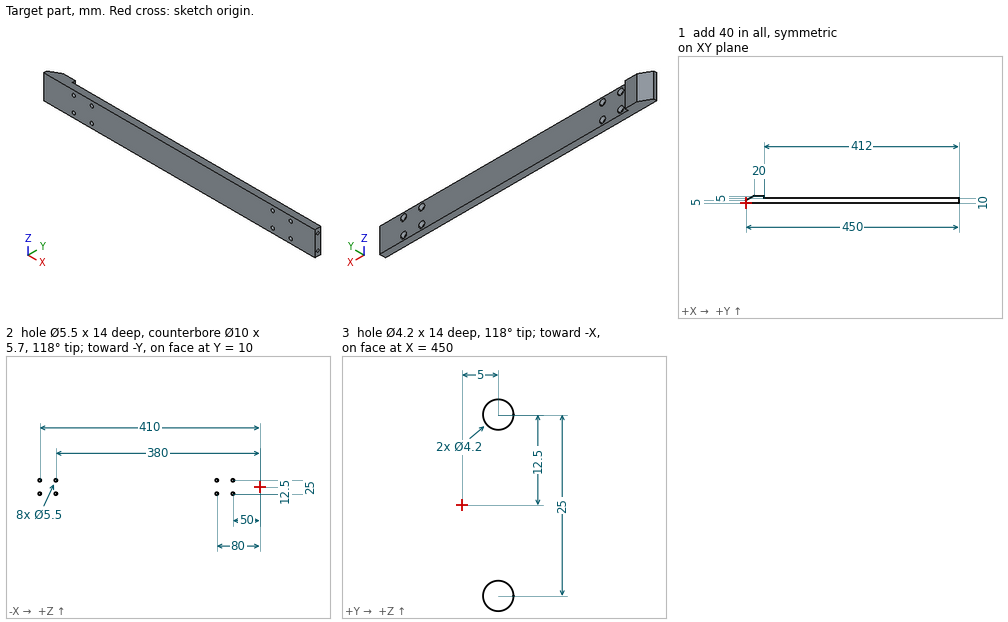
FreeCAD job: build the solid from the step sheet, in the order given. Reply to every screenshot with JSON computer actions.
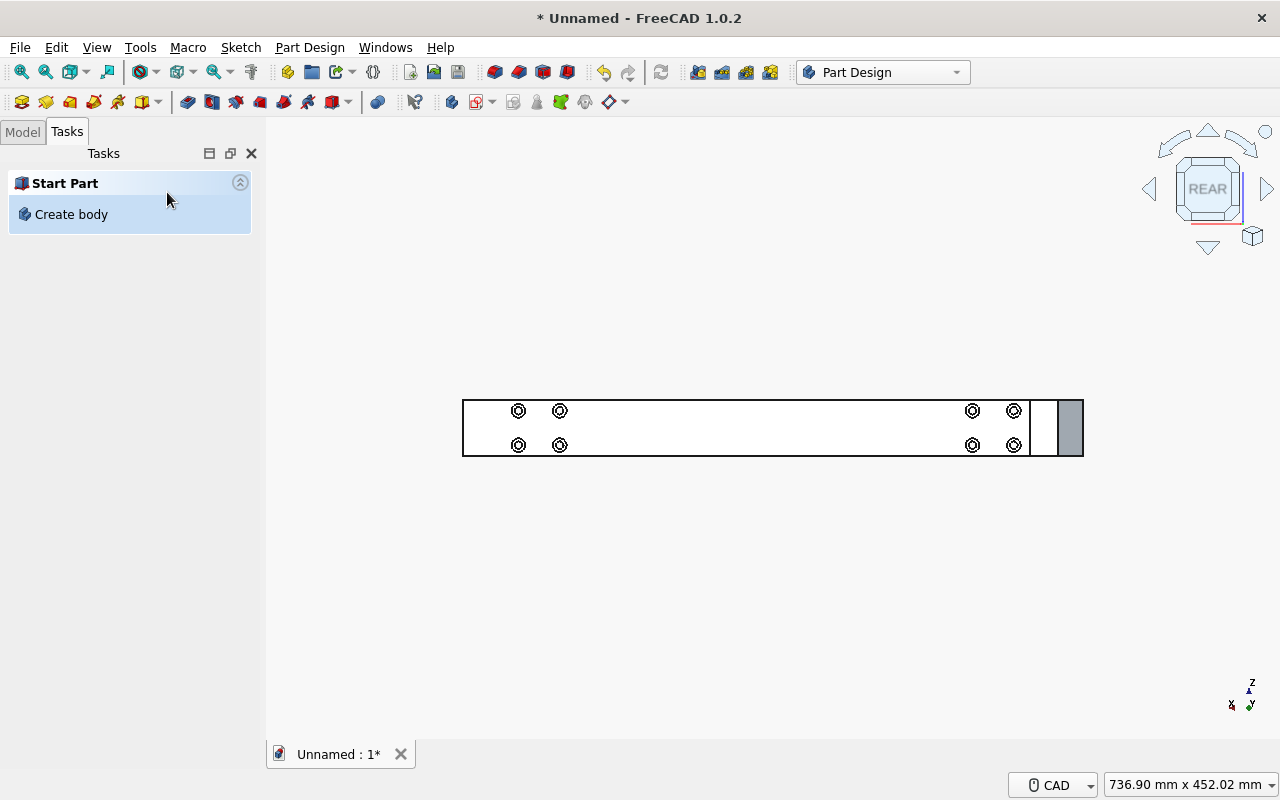
{"action": "key", "text": "0"}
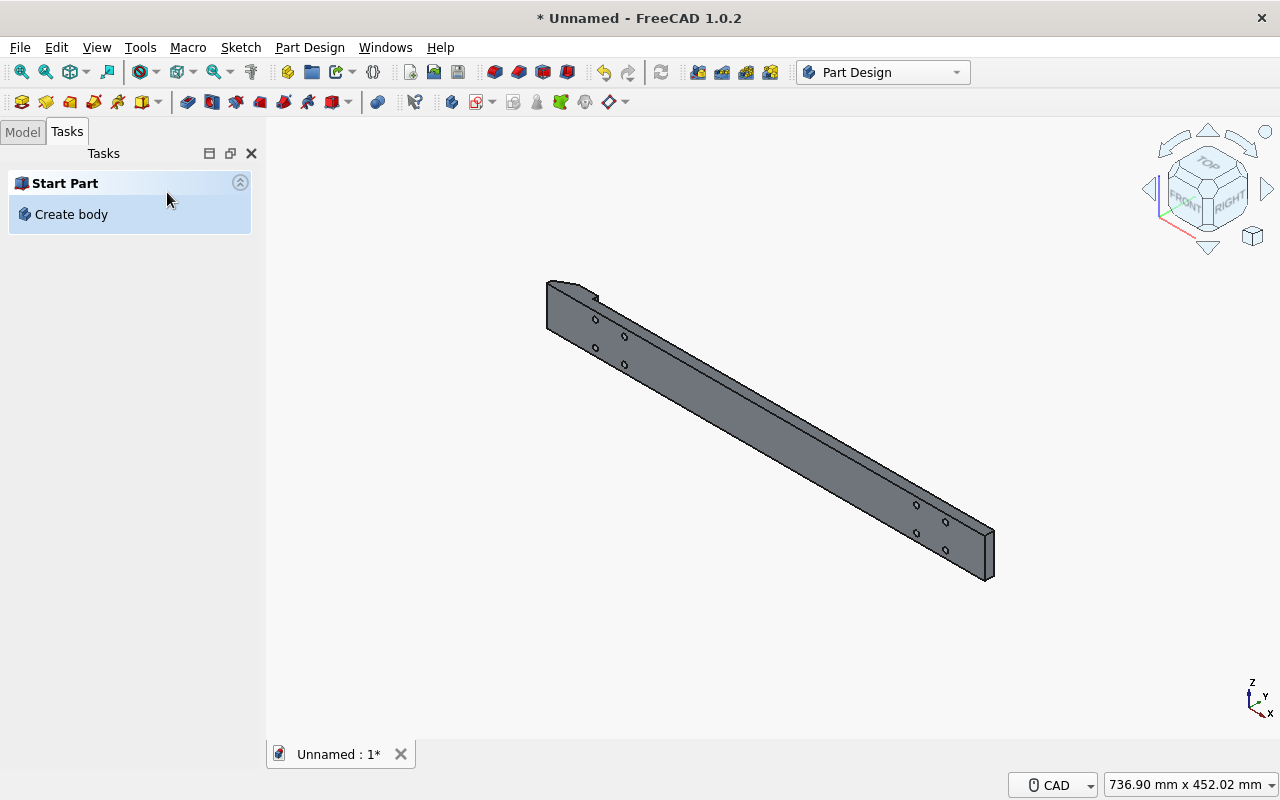
{"action": "scroll", "coordinate": [989, 542], "scroll_direction": "up", "scroll_amount": 3}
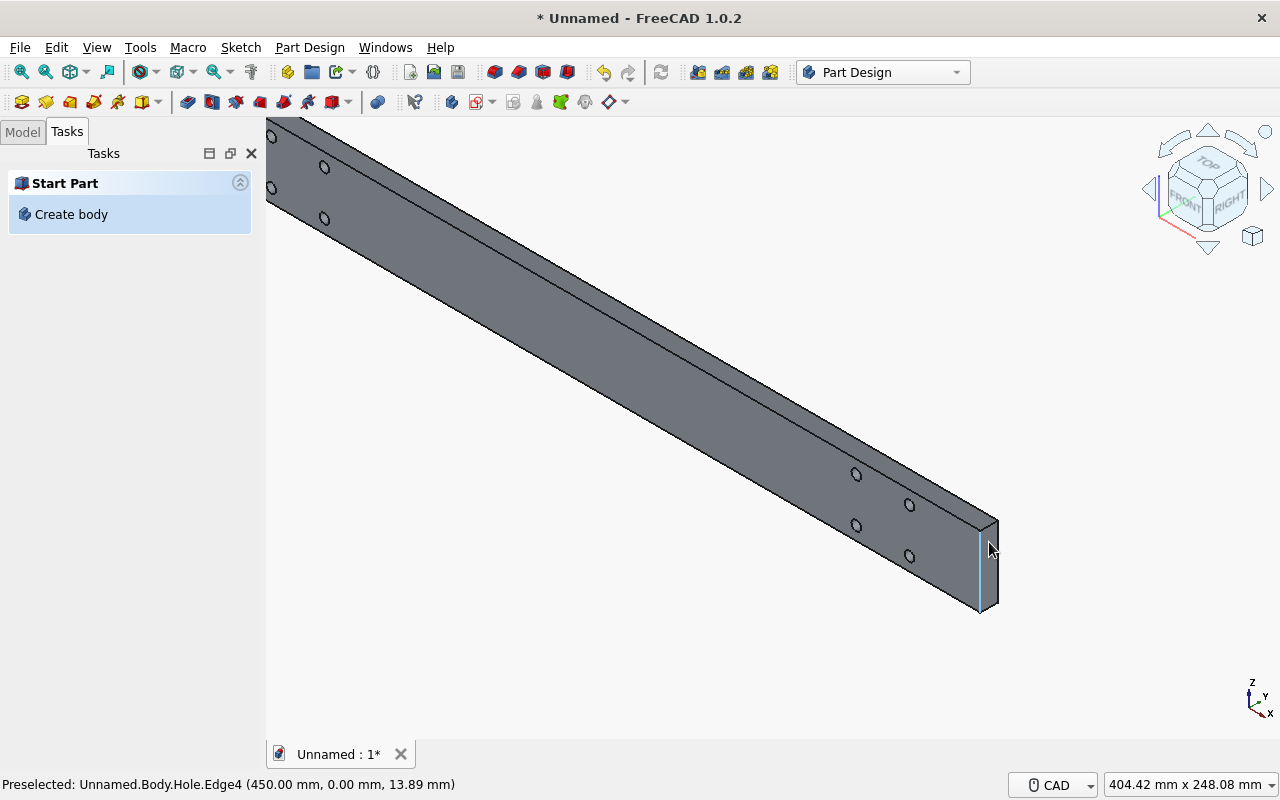
{"action": "left_click", "coordinate": [989, 542]}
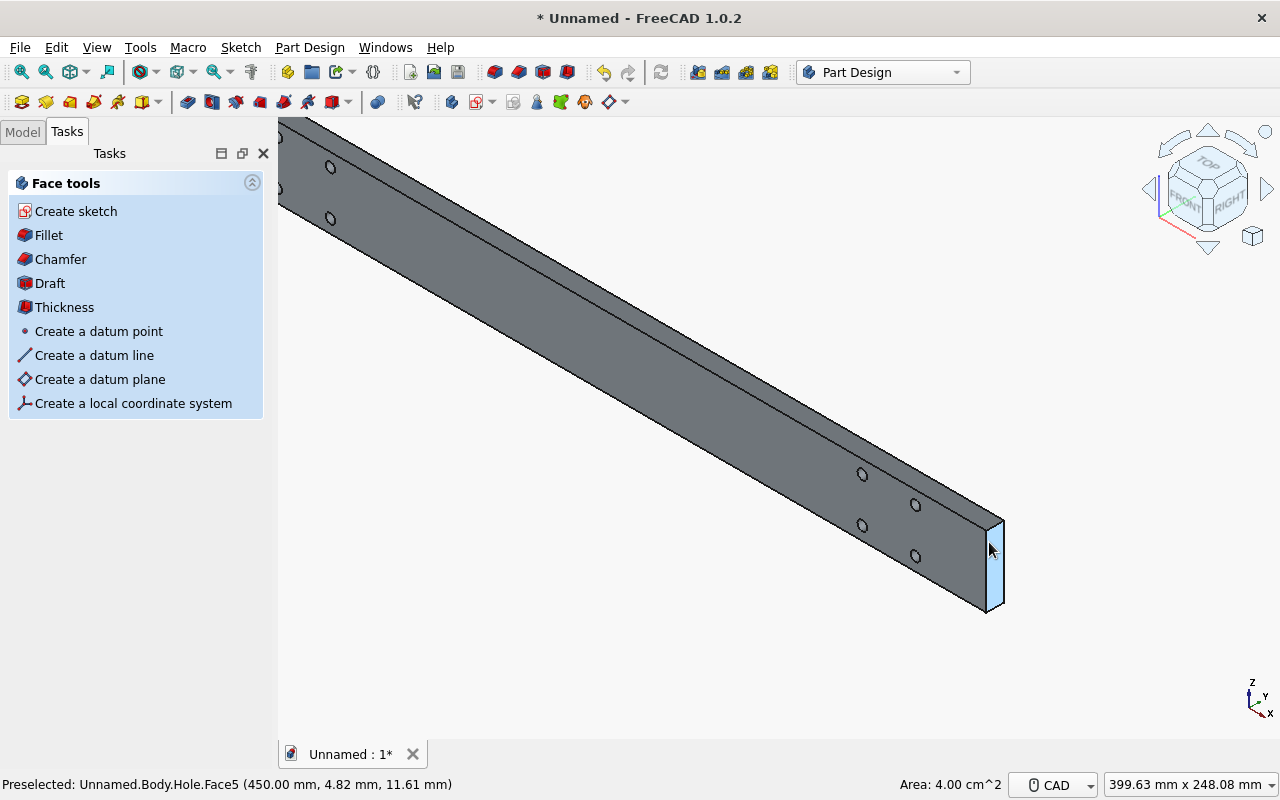
{"action": "left_click", "coordinate": [476, 102]}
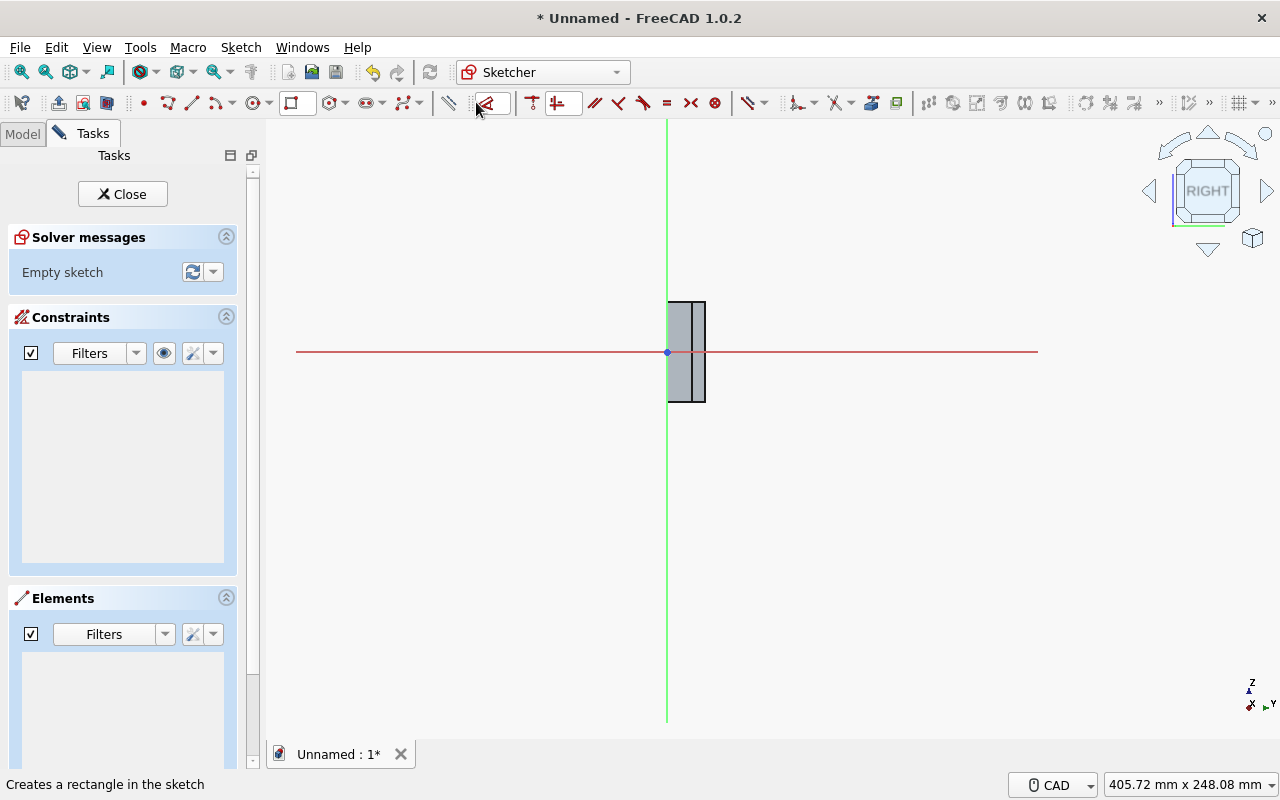
{"action": "scroll", "coordinate": [669, 333], "scroll_direction": "up", "scroll_amount": 8}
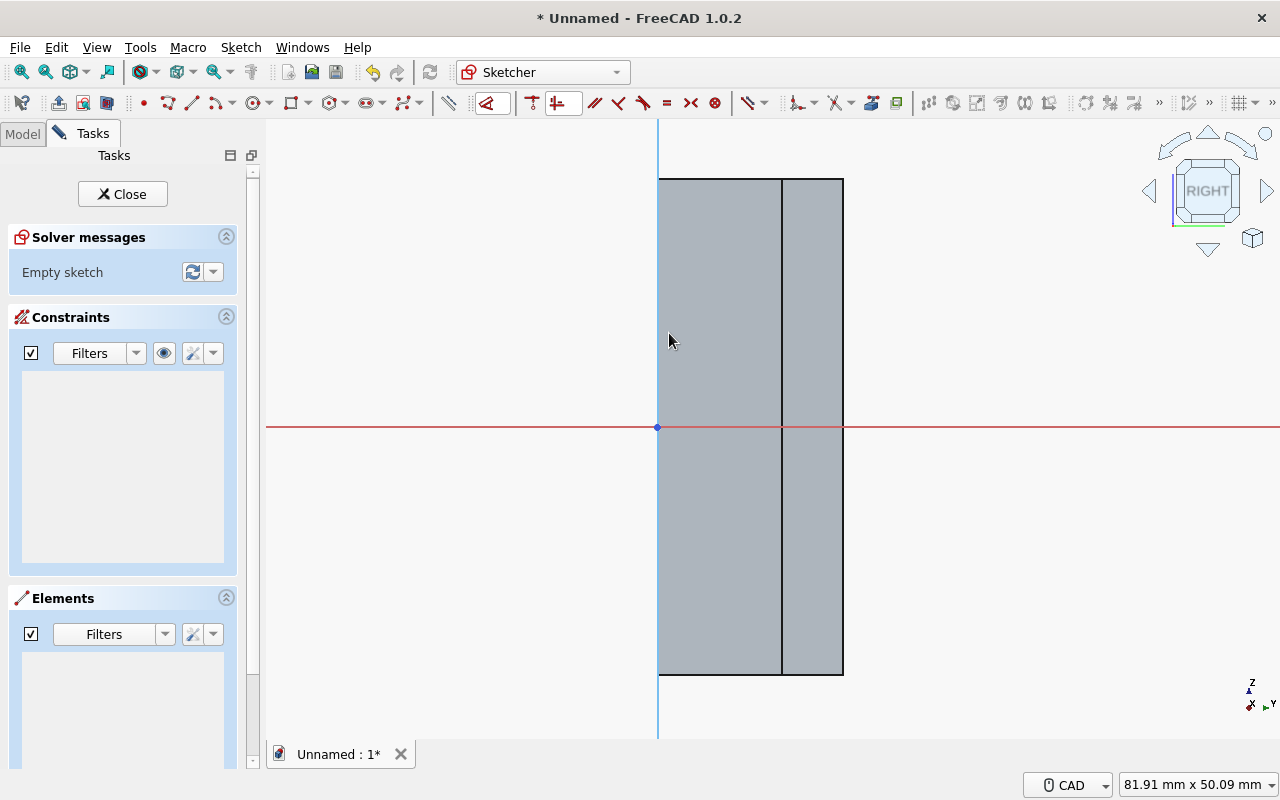
{"action": "left_click", "coordinate": [254, 104]}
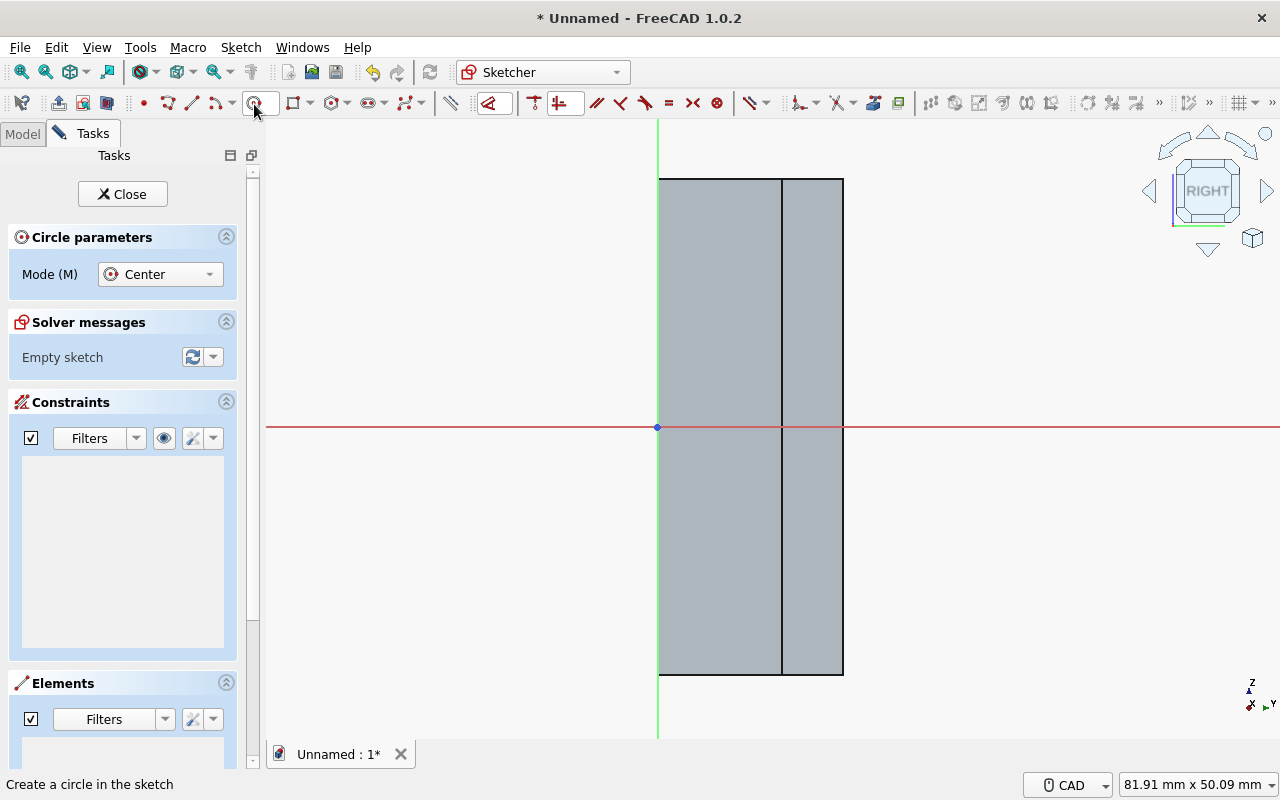
{"action": "left_click", "coordinate": [720, 272]}
{"action": "left_click", "coordinate": [738, 254]}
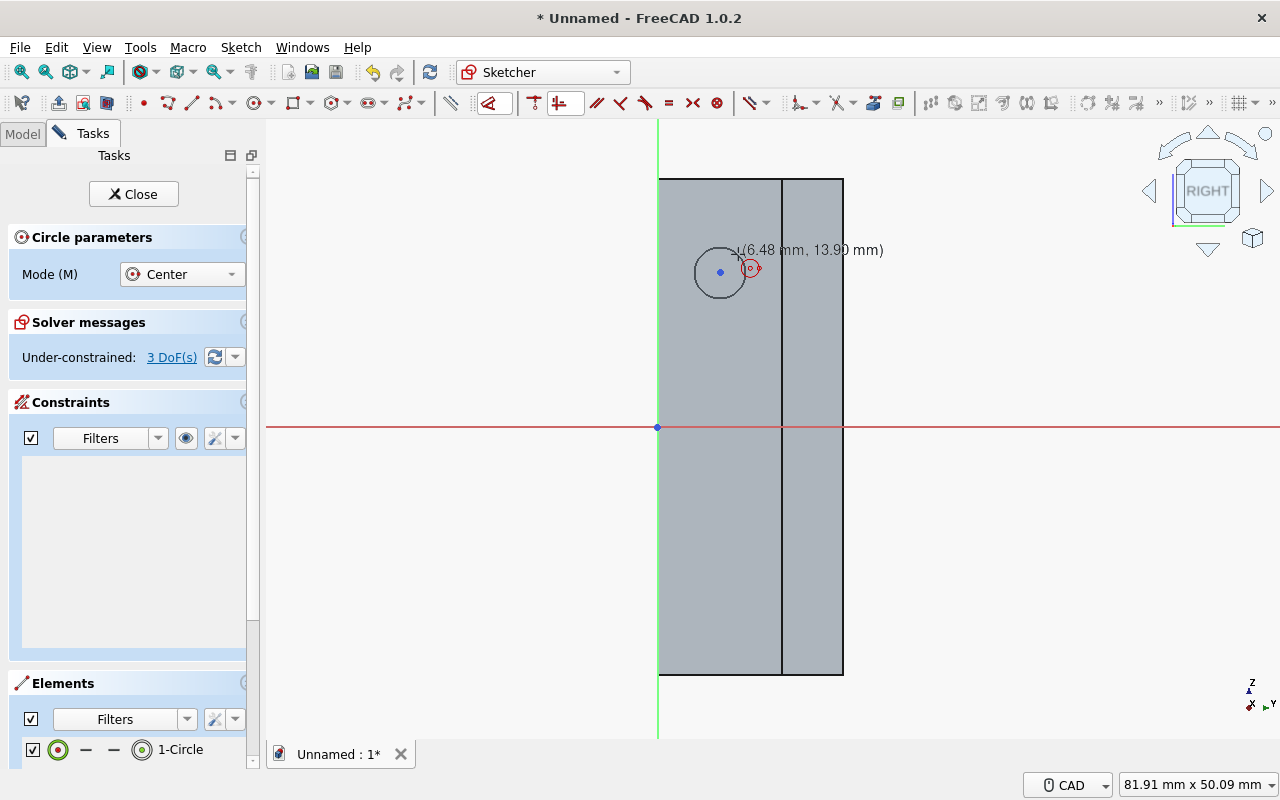
{"action": "left_click", "coordinate": [720, 582]}
{"action": "left_click", "coordinate": [738, 563]}
{"action": "key", "text": "Escape"}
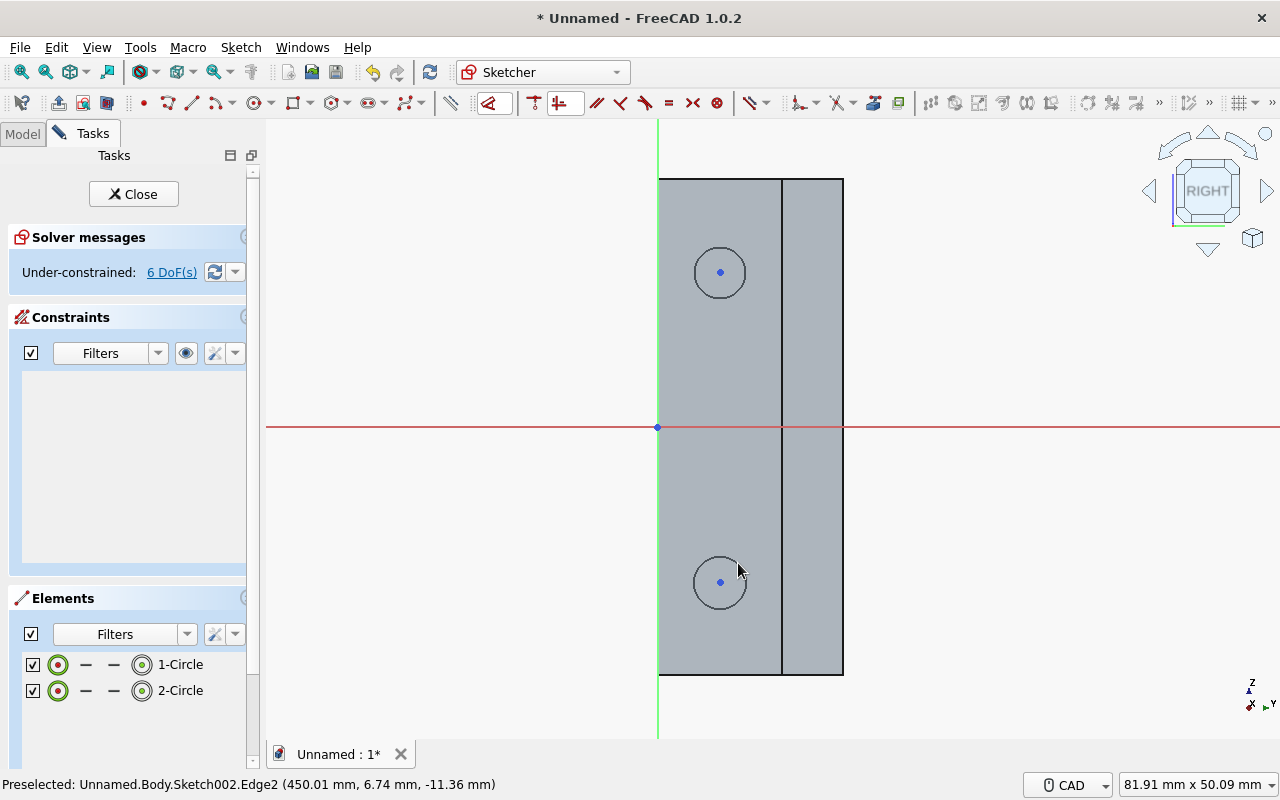
{"action": "left_click", "coordinate": [738, 255]}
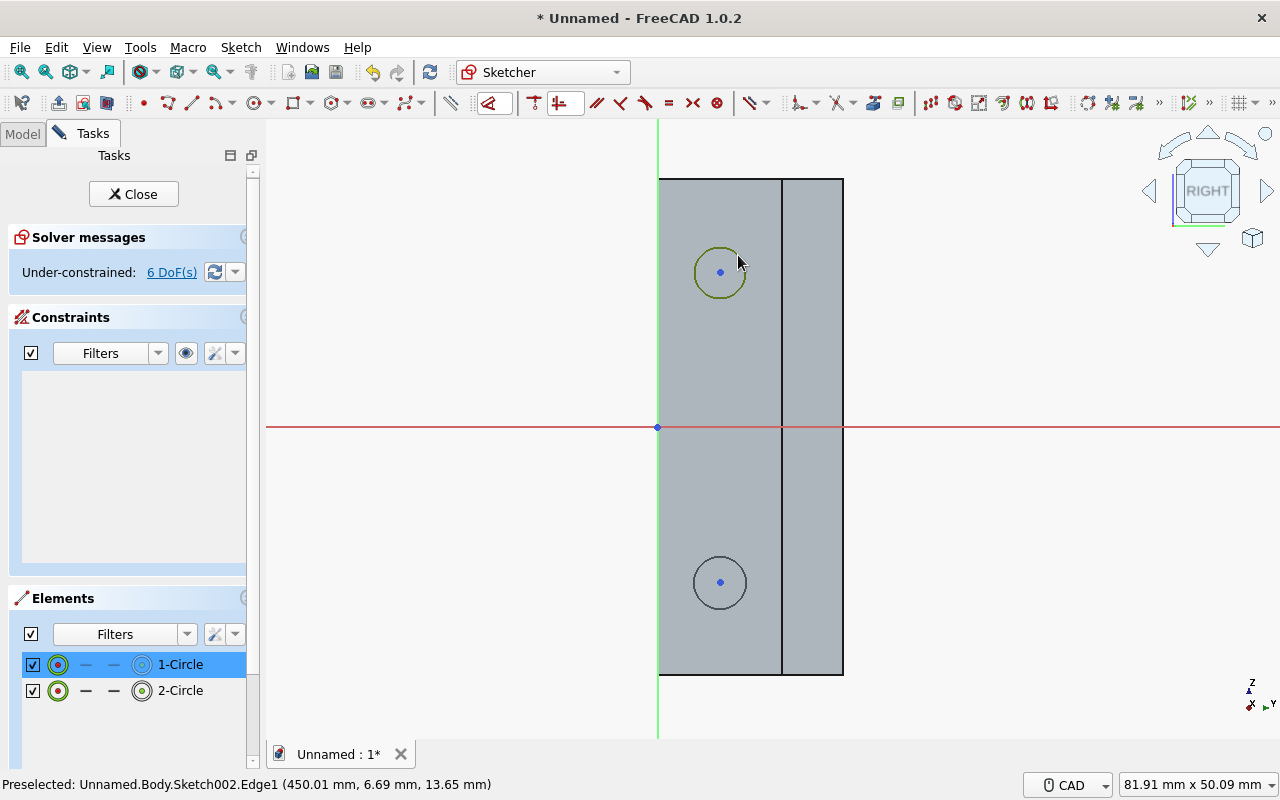
{"action": "left_click", "coordinate": [738, 564]}